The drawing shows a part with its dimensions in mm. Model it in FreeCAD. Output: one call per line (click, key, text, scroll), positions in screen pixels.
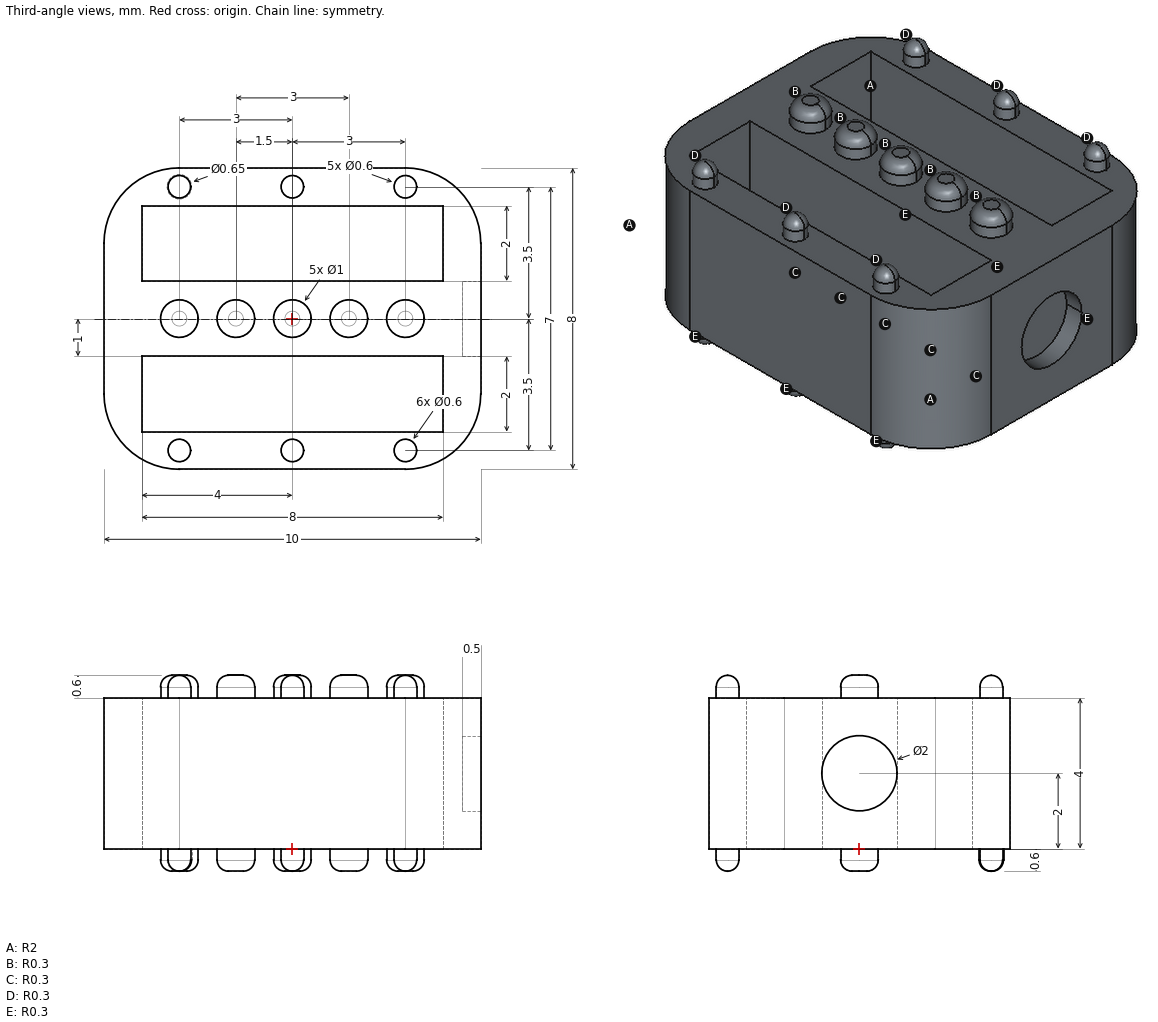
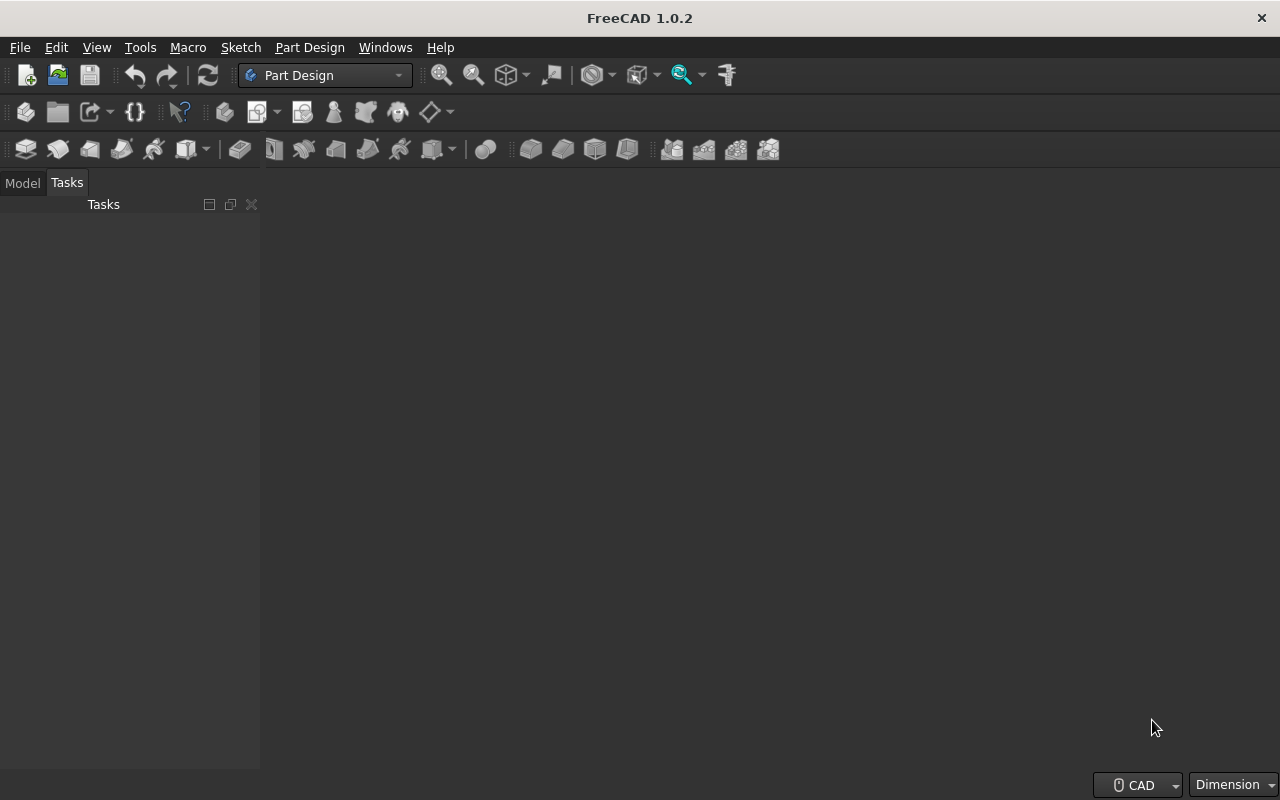
key(ctrl+n)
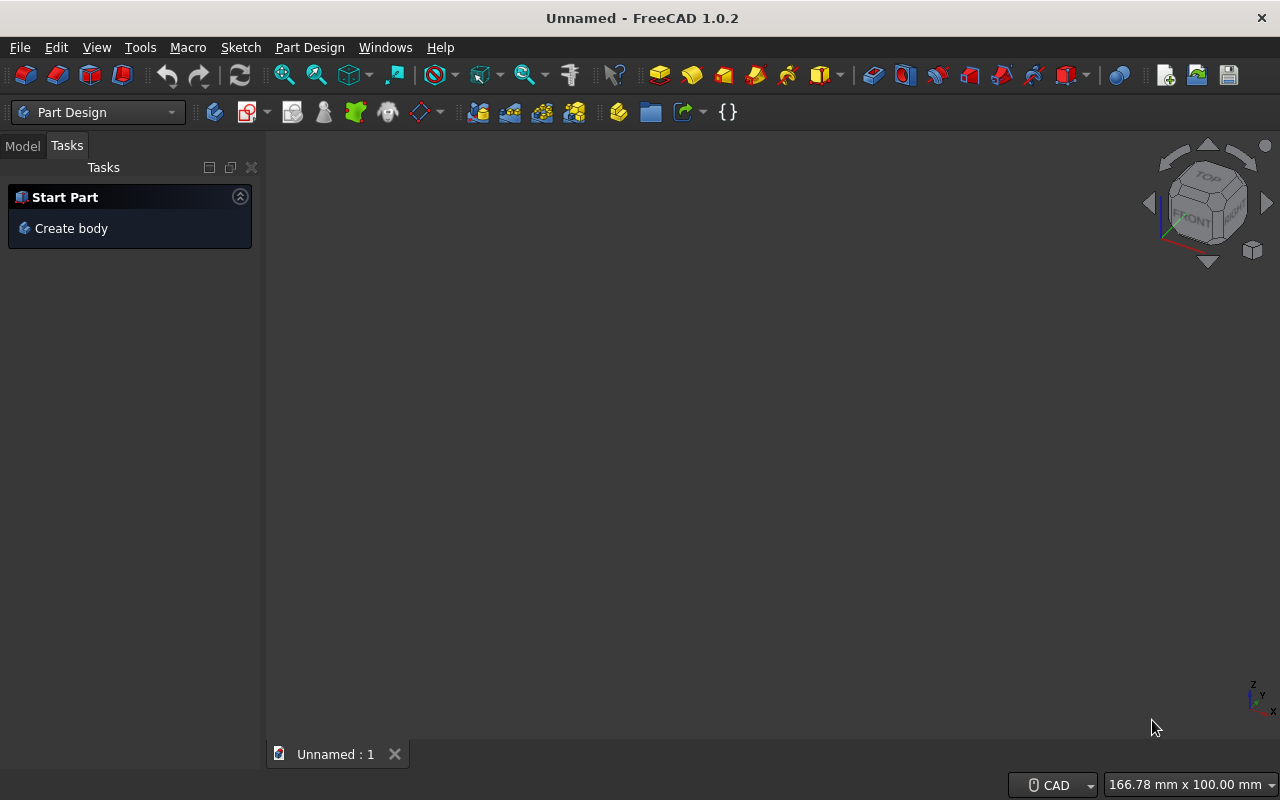
click(248, 112)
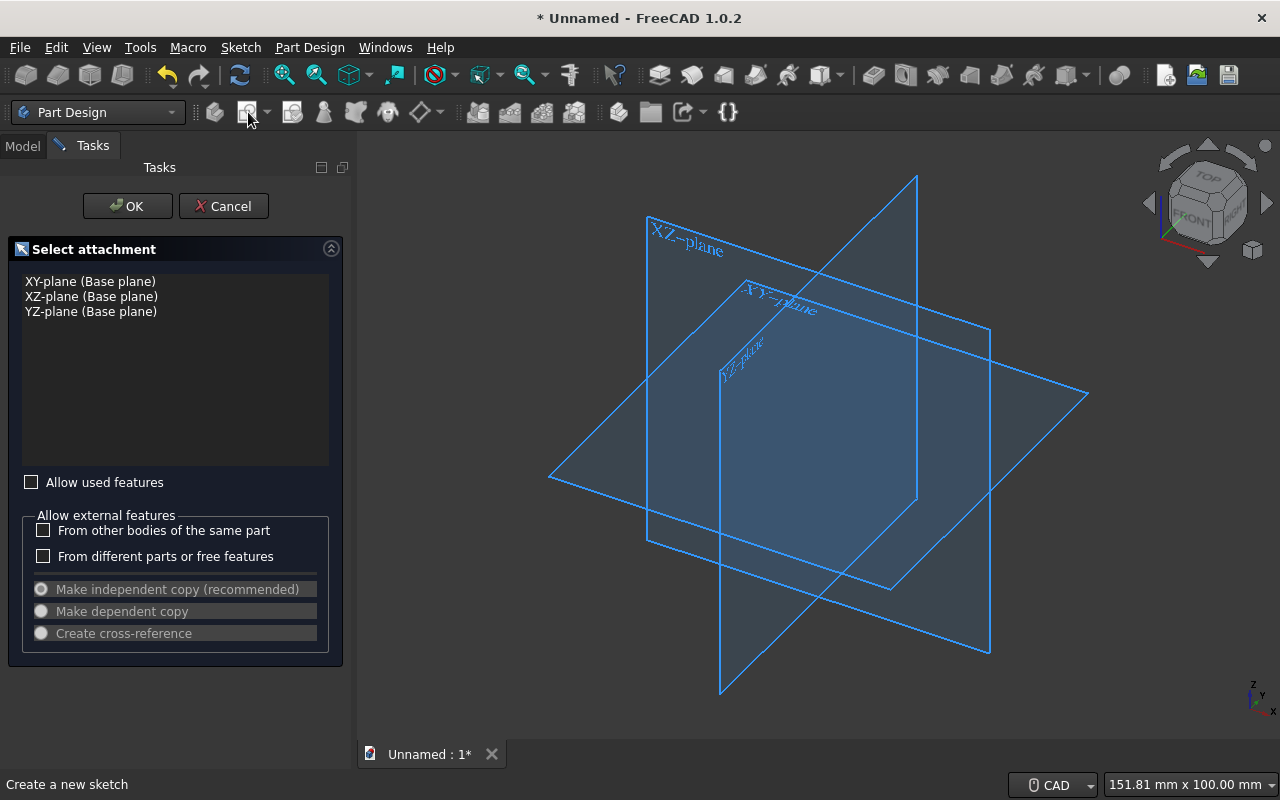
click(82, 282)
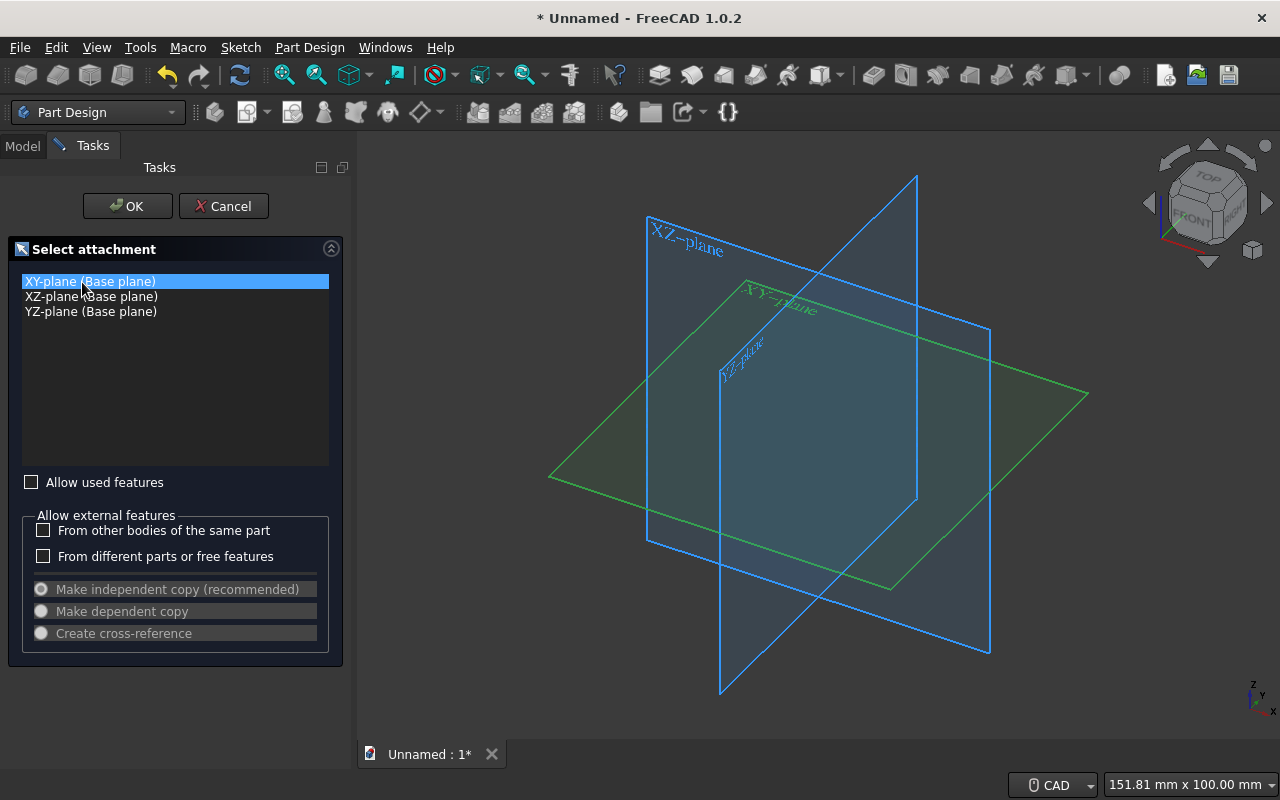
click(128, 206)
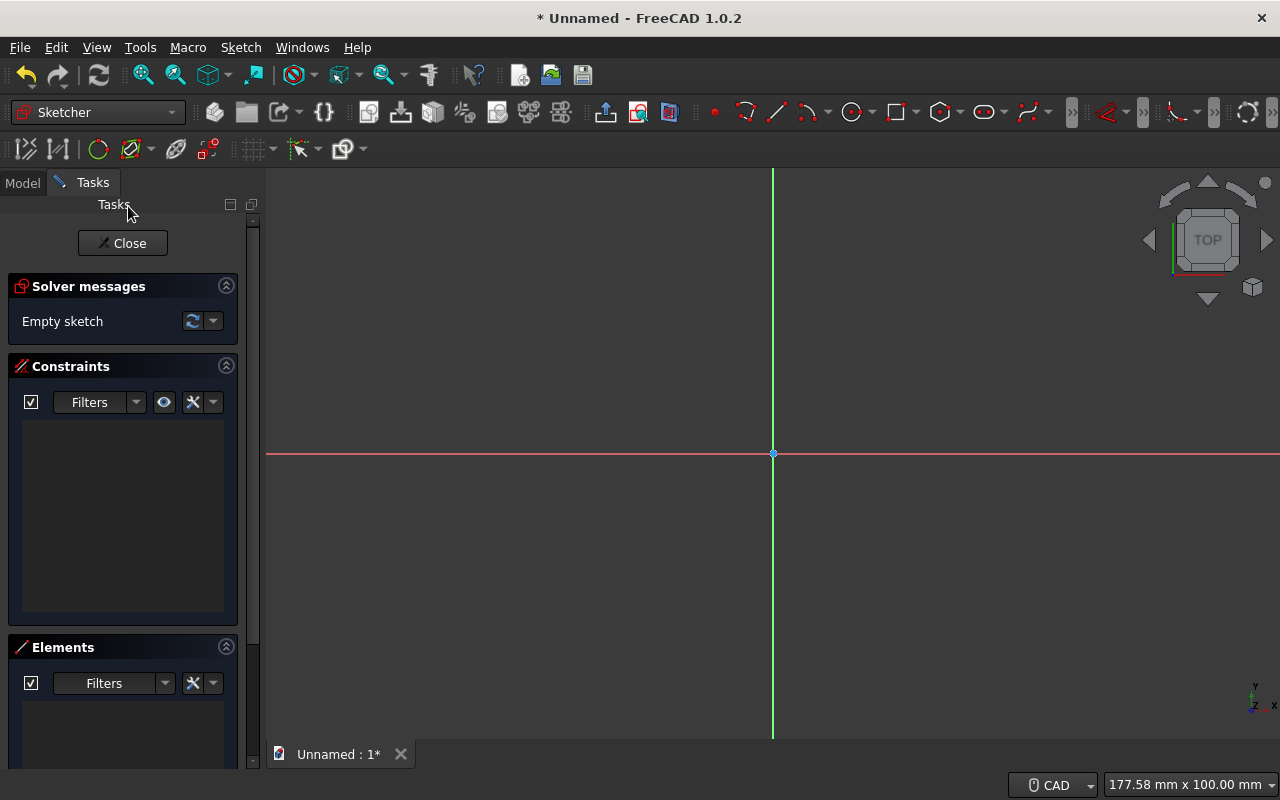
scroll(784, 454, up, 10)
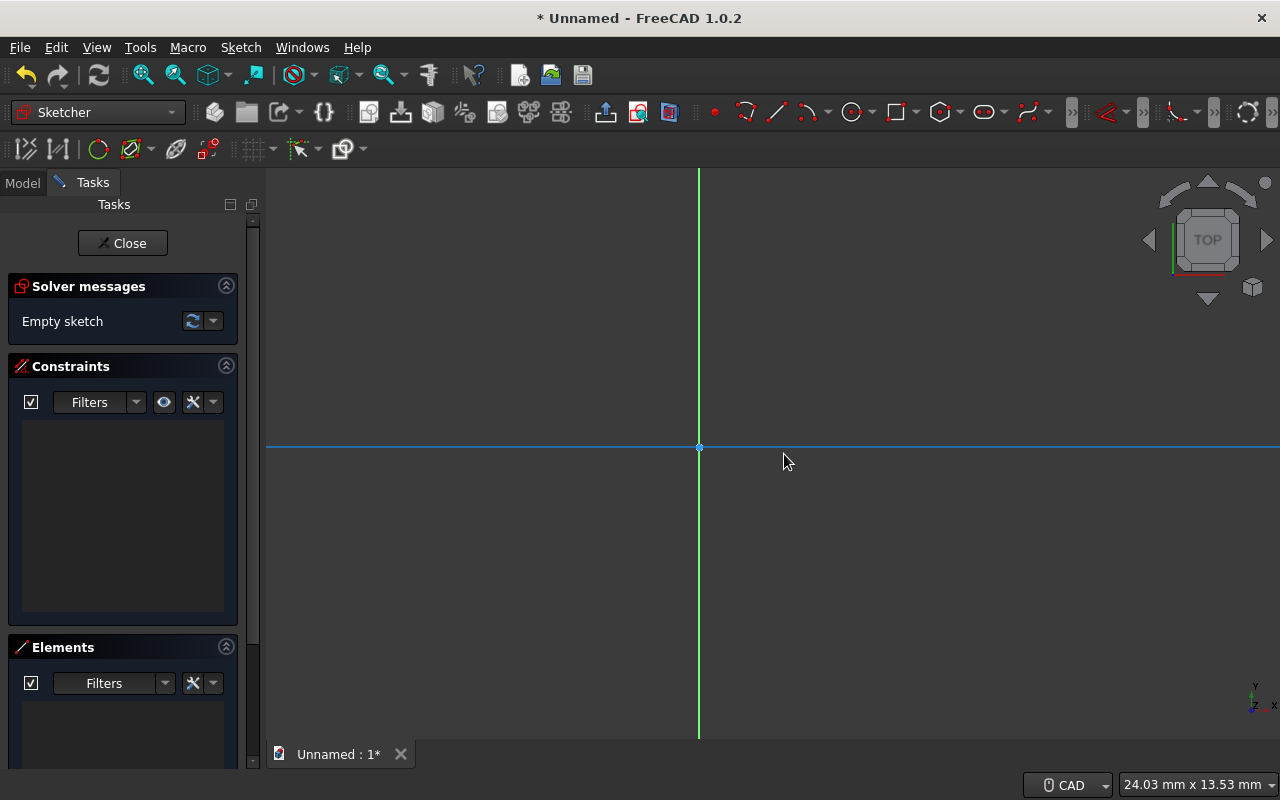
key(g)
key(v)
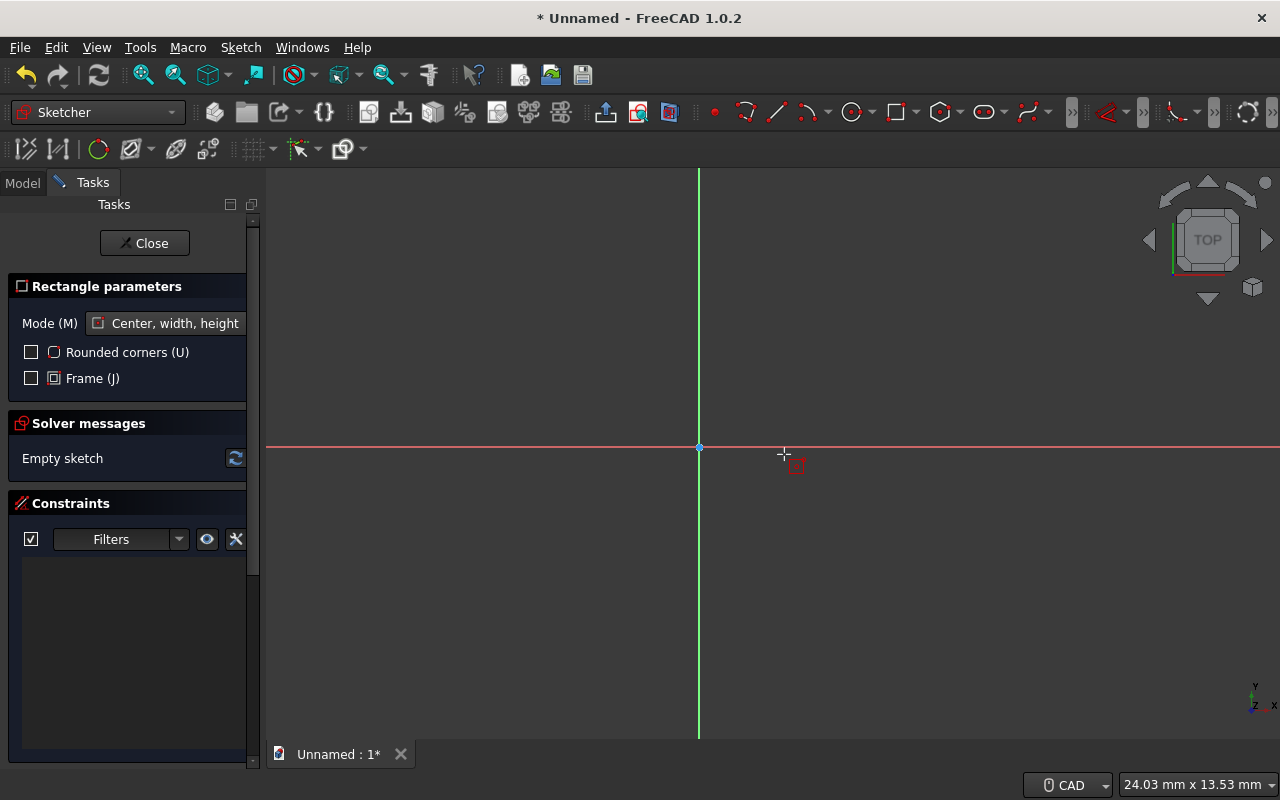
click(699, 447)
move(910, 278)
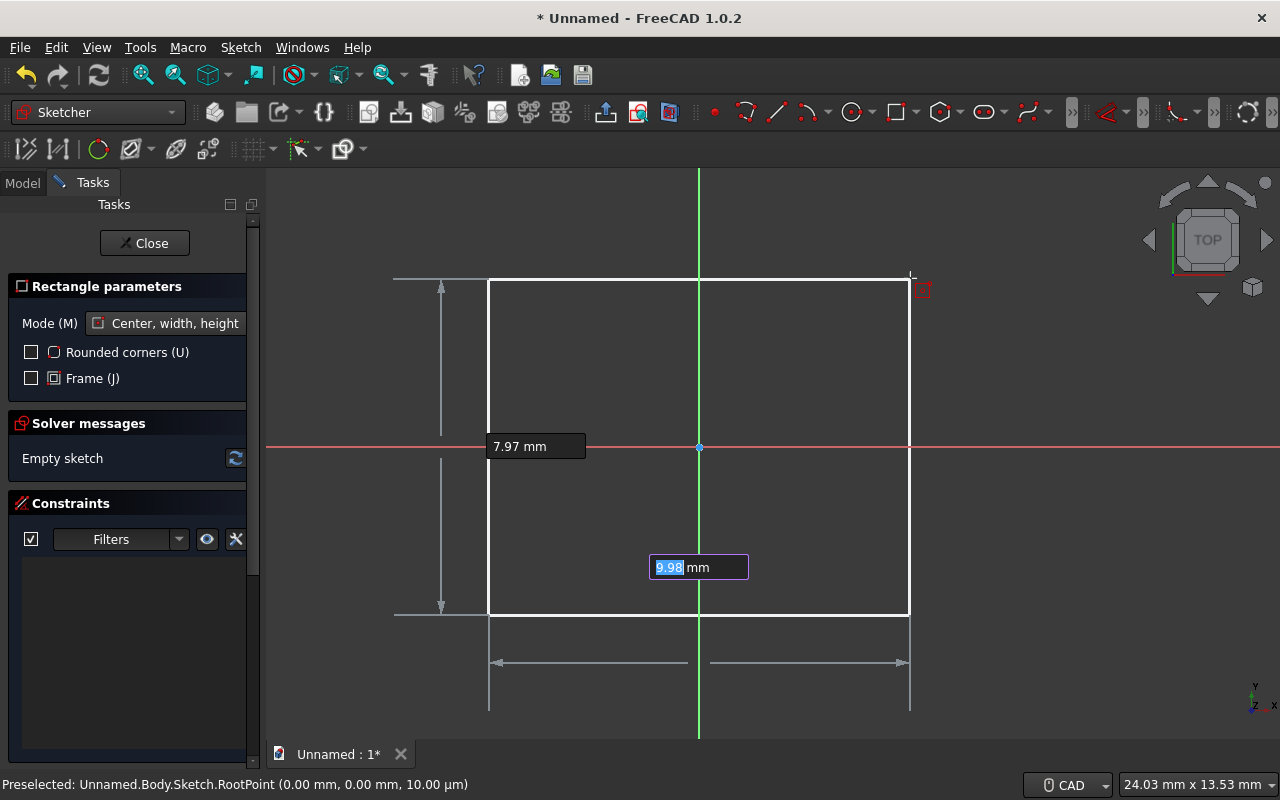
text(10)
key(Tab)
text(8)
key(Return)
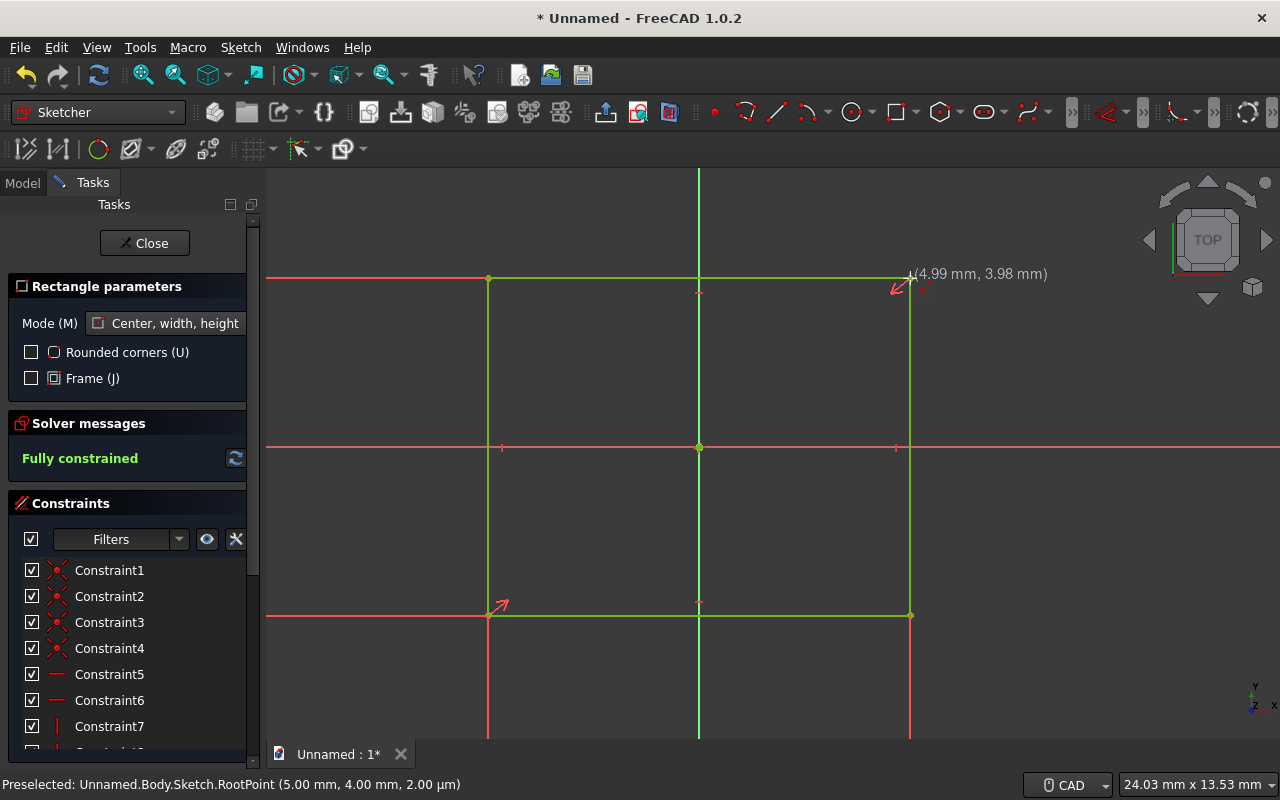
click(896, 112)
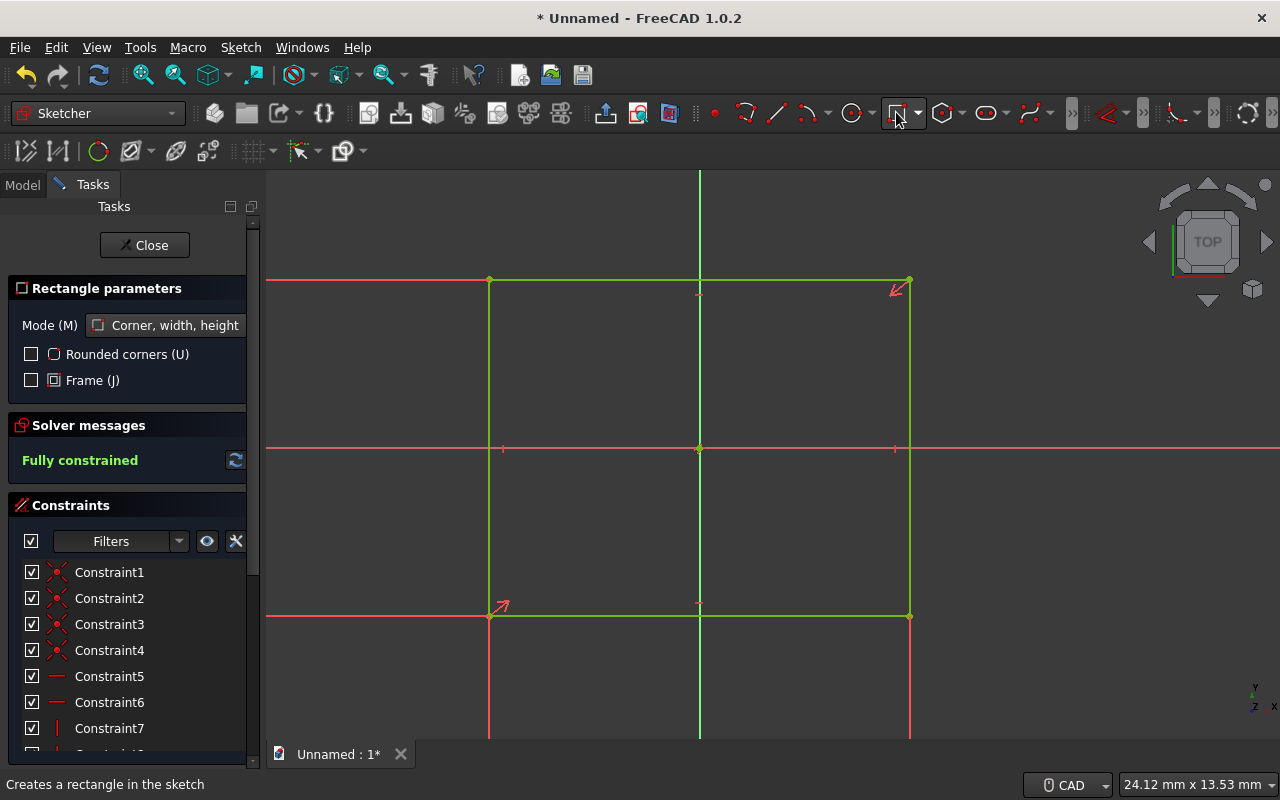
click(532, 490)
move(868, 574)